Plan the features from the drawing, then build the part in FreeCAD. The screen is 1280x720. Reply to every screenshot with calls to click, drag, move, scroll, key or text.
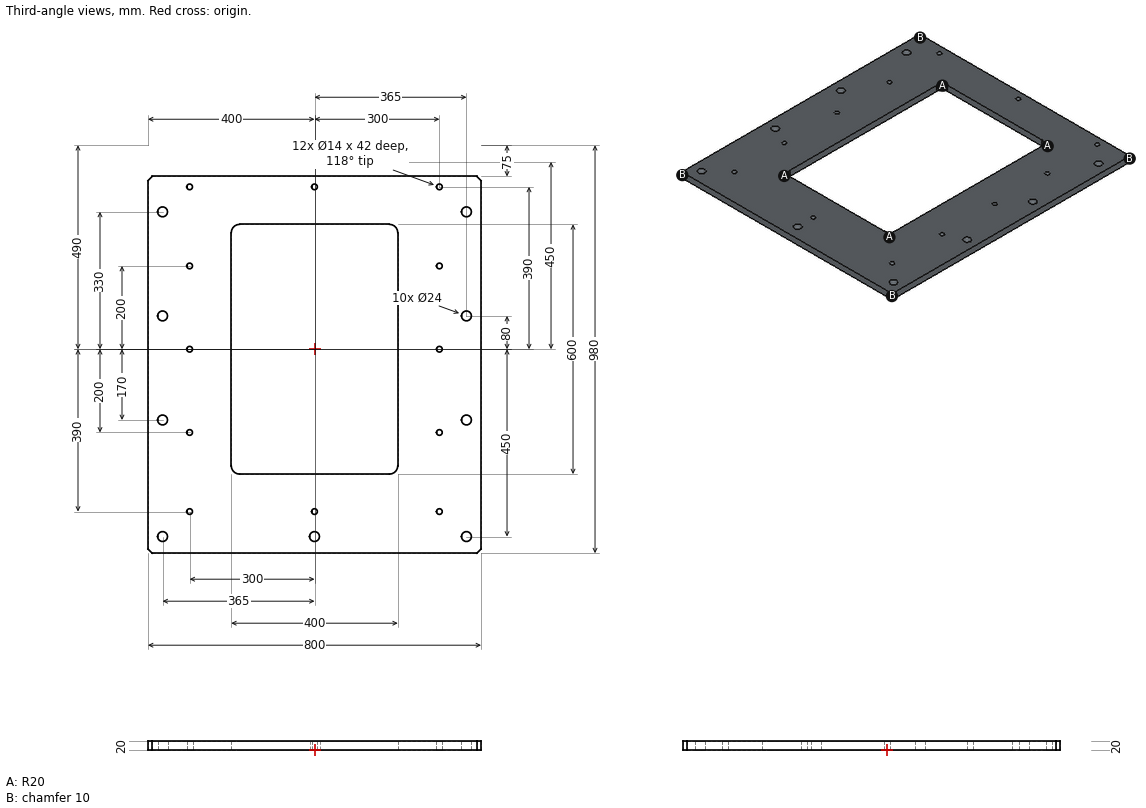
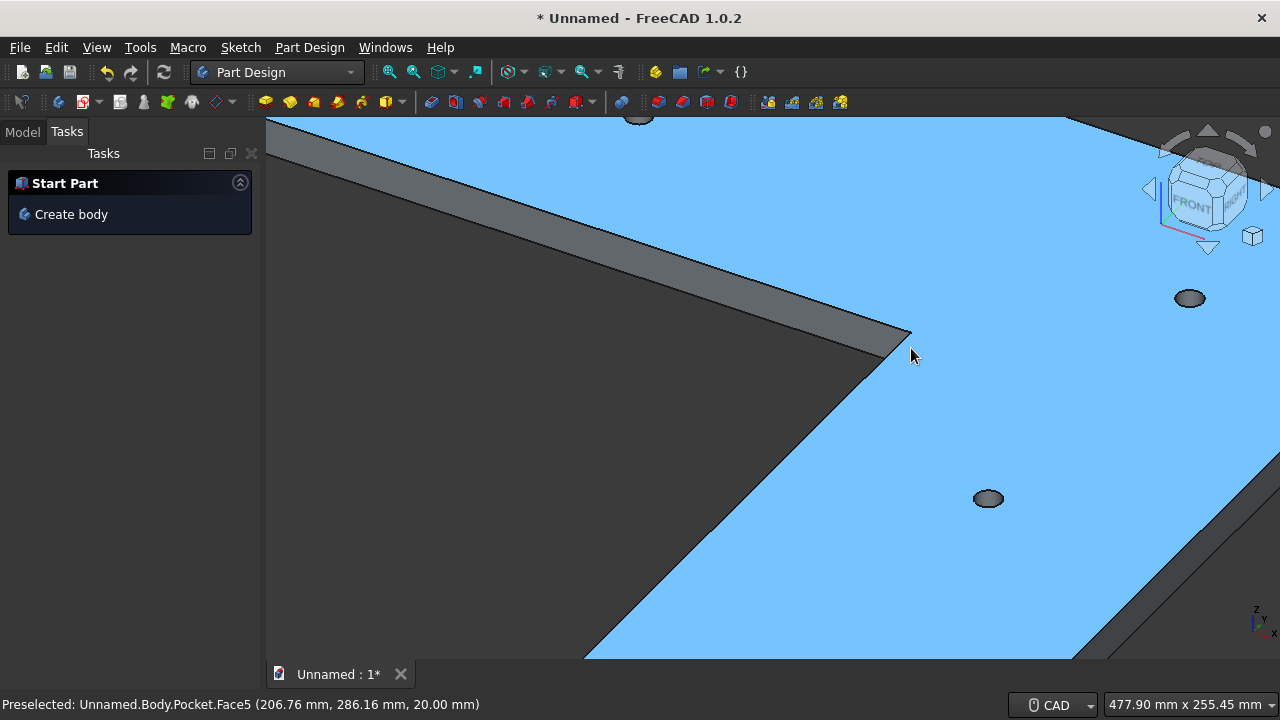
click(390, 72)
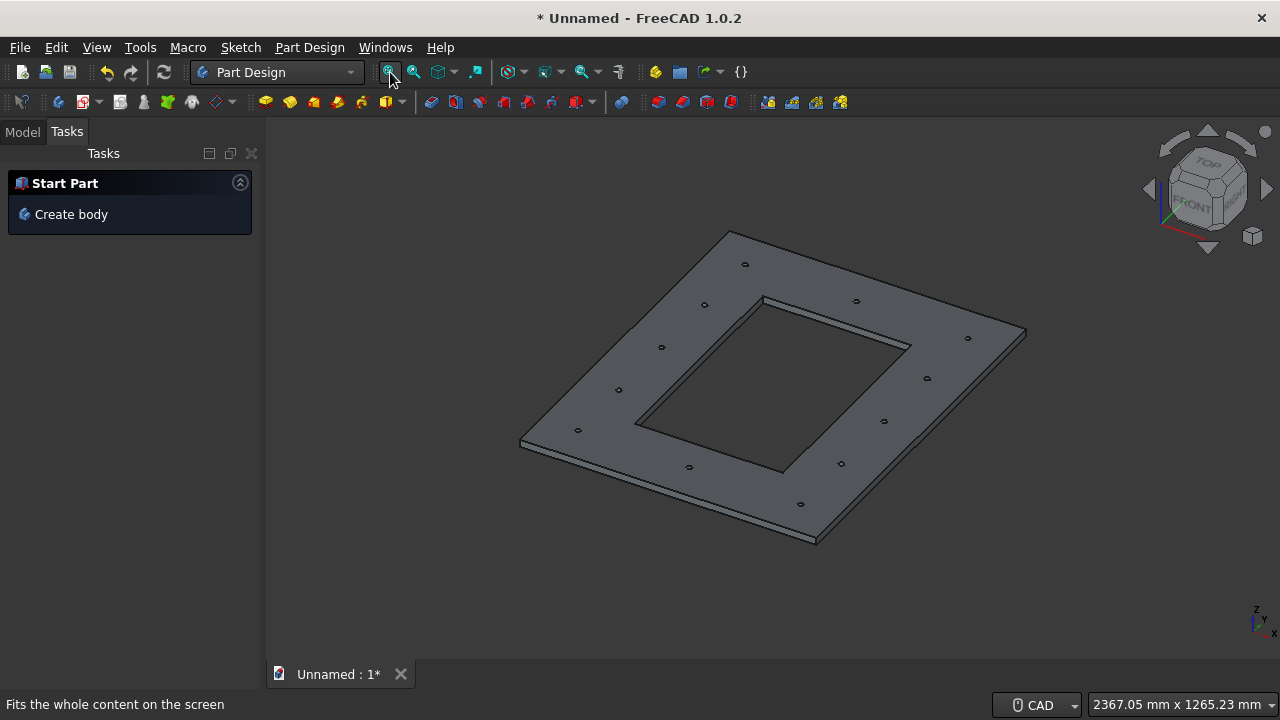
key(0)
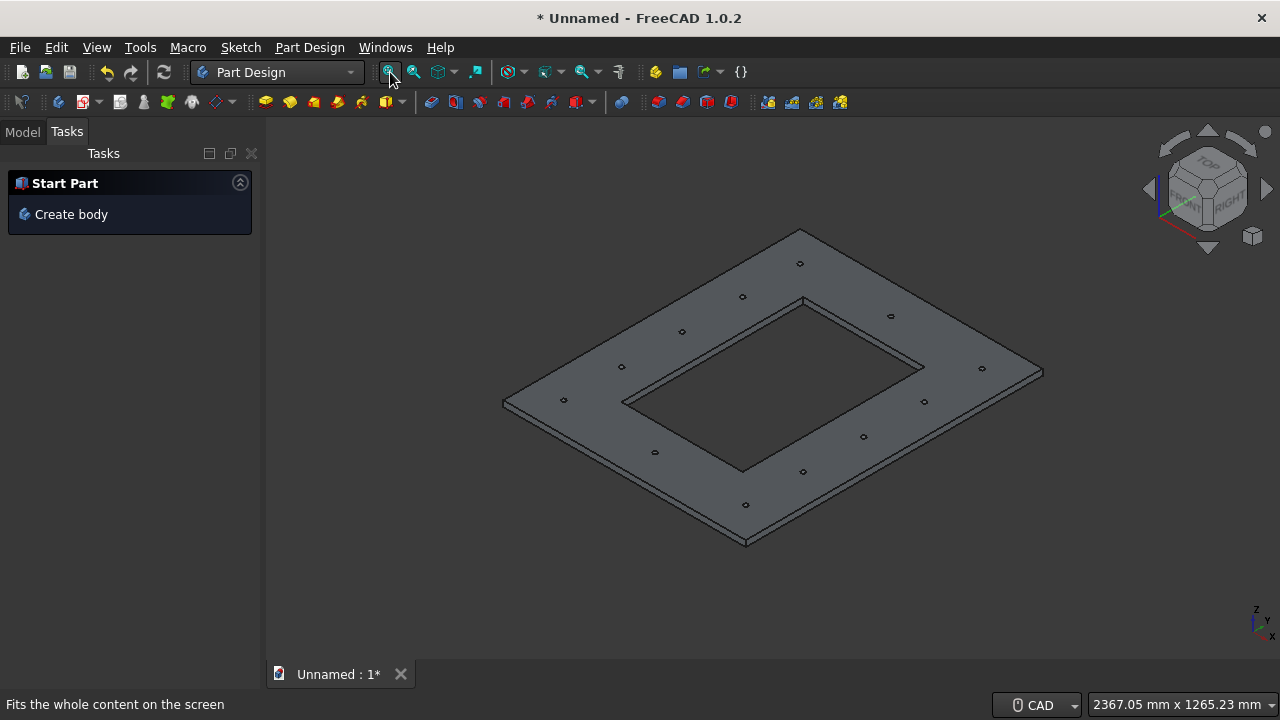
scroll(924, 370, up, 8)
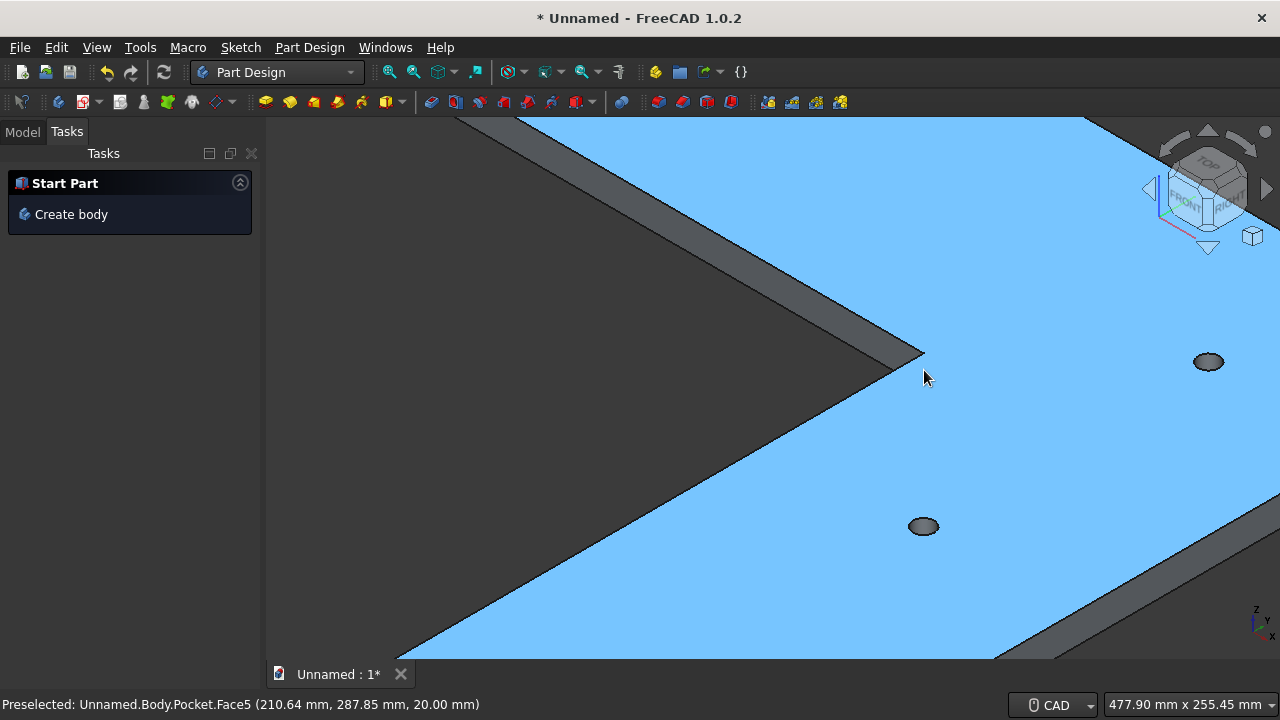
click(390, 72)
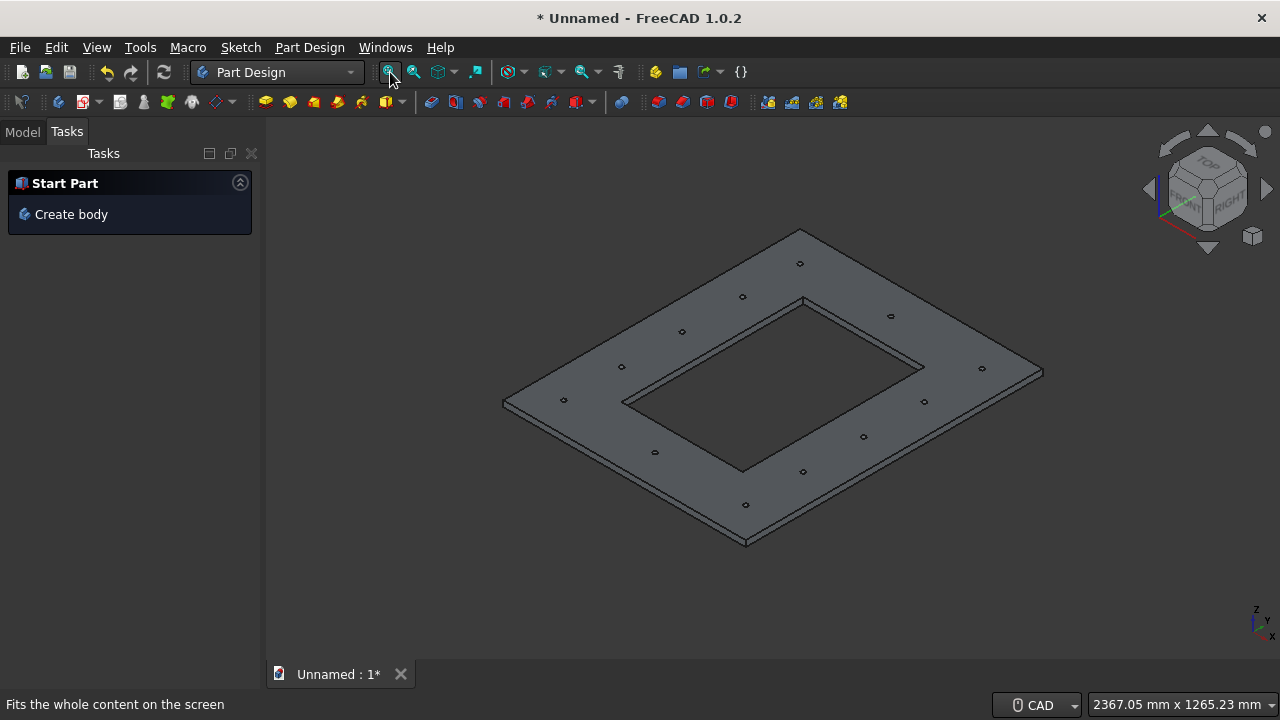
key(2)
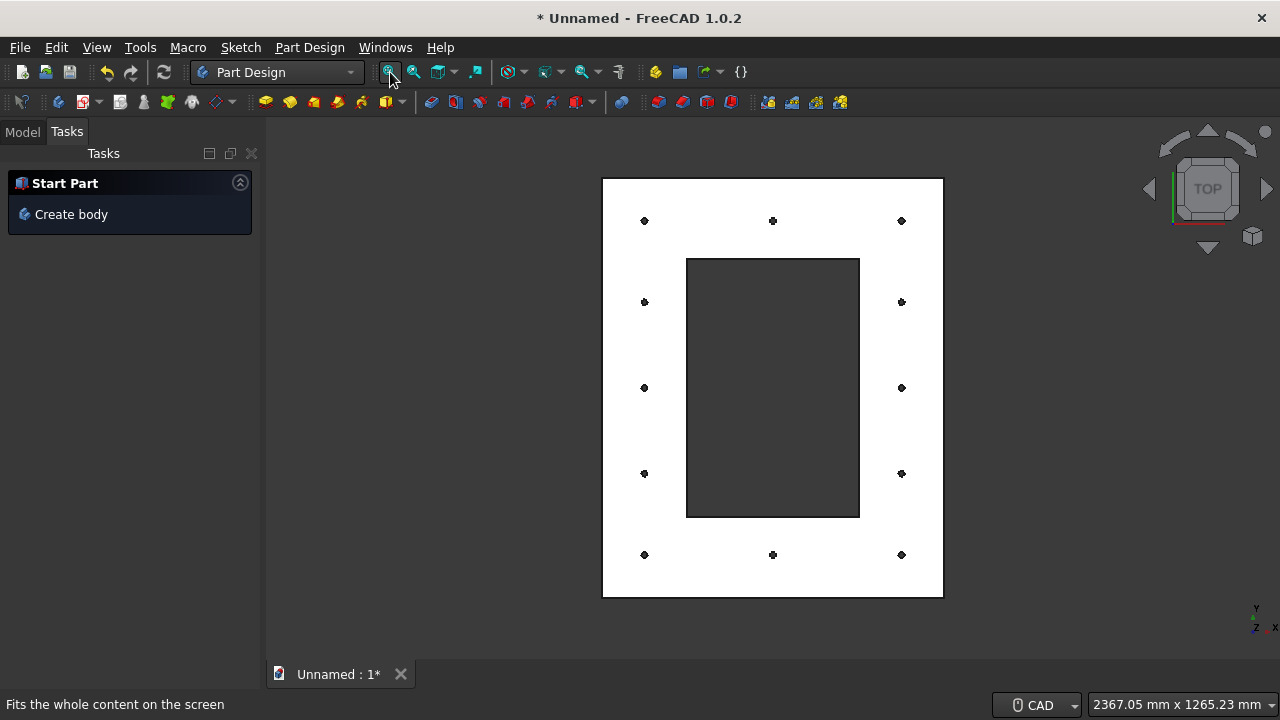
scroll(859, 258, up, 8)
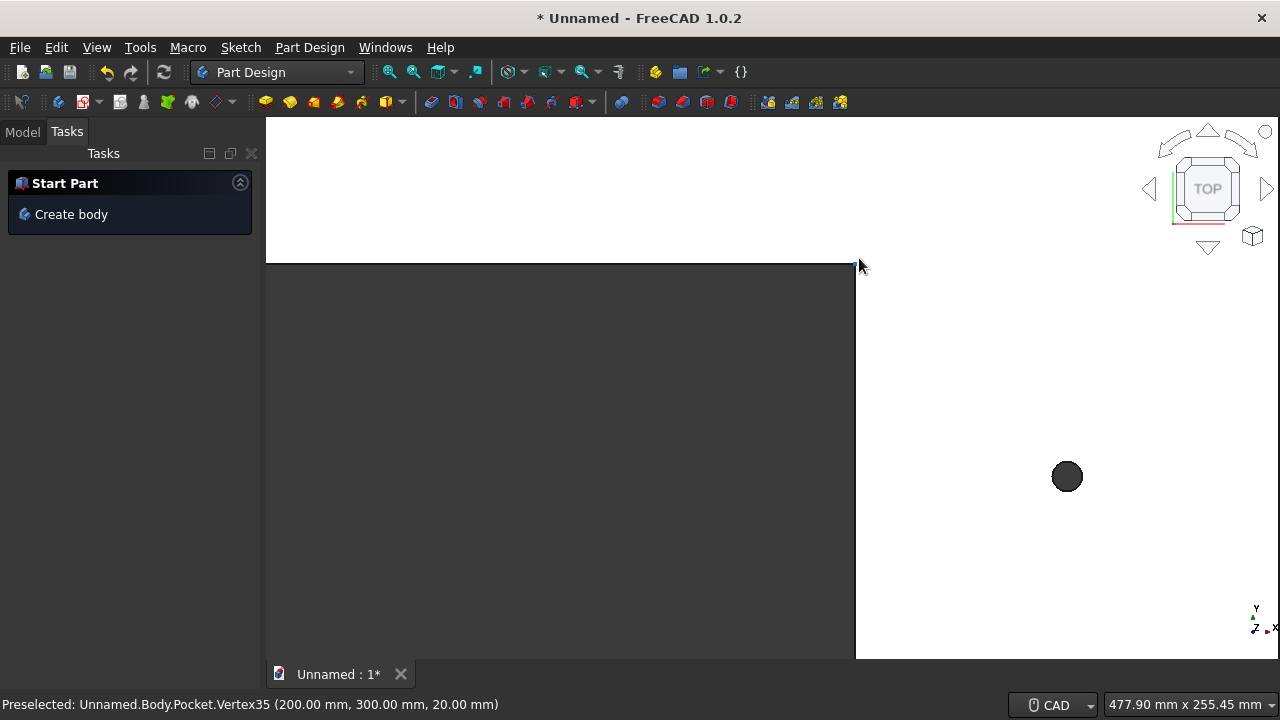
click(390, 72)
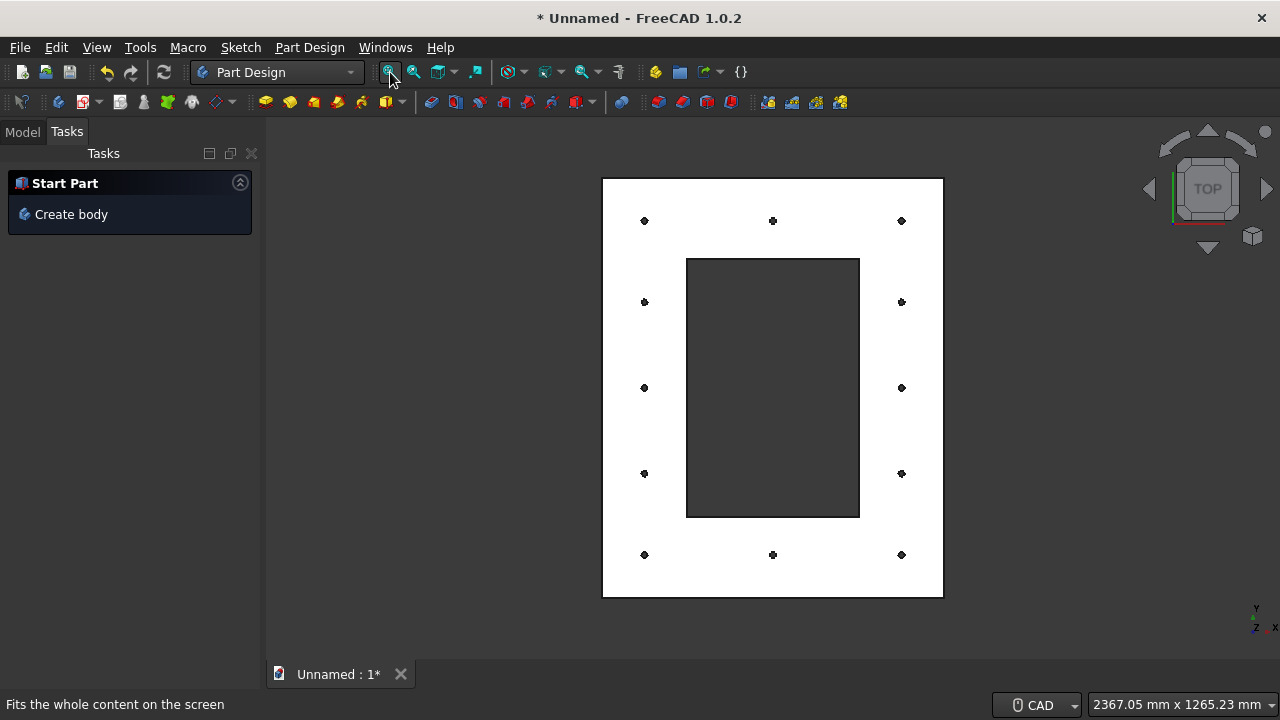
key(1)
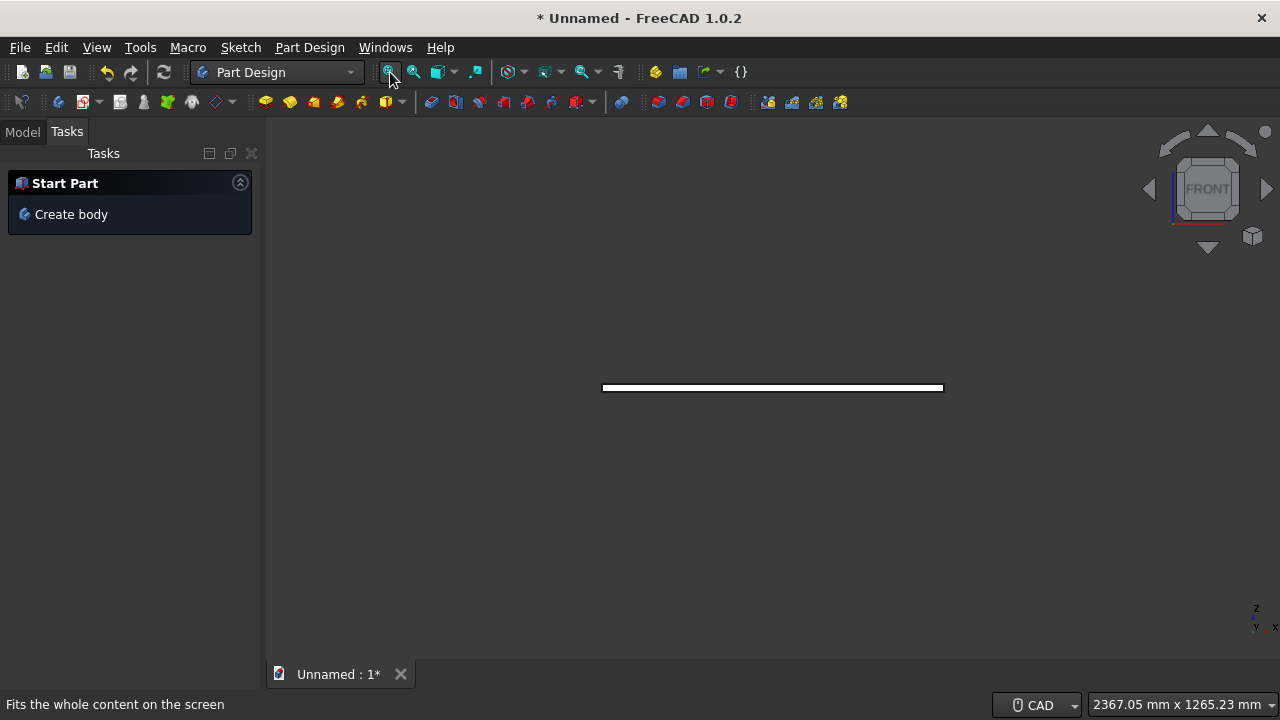
click(390, 72)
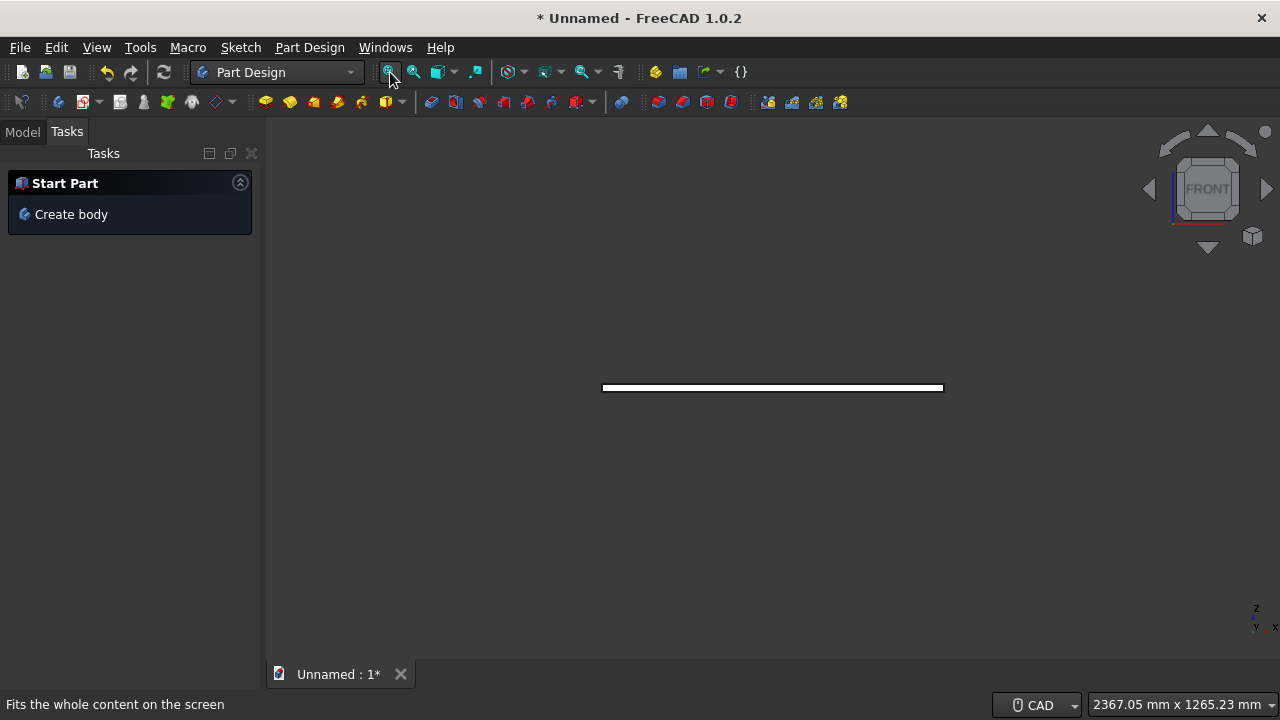
scroll(859, 387, up, 8)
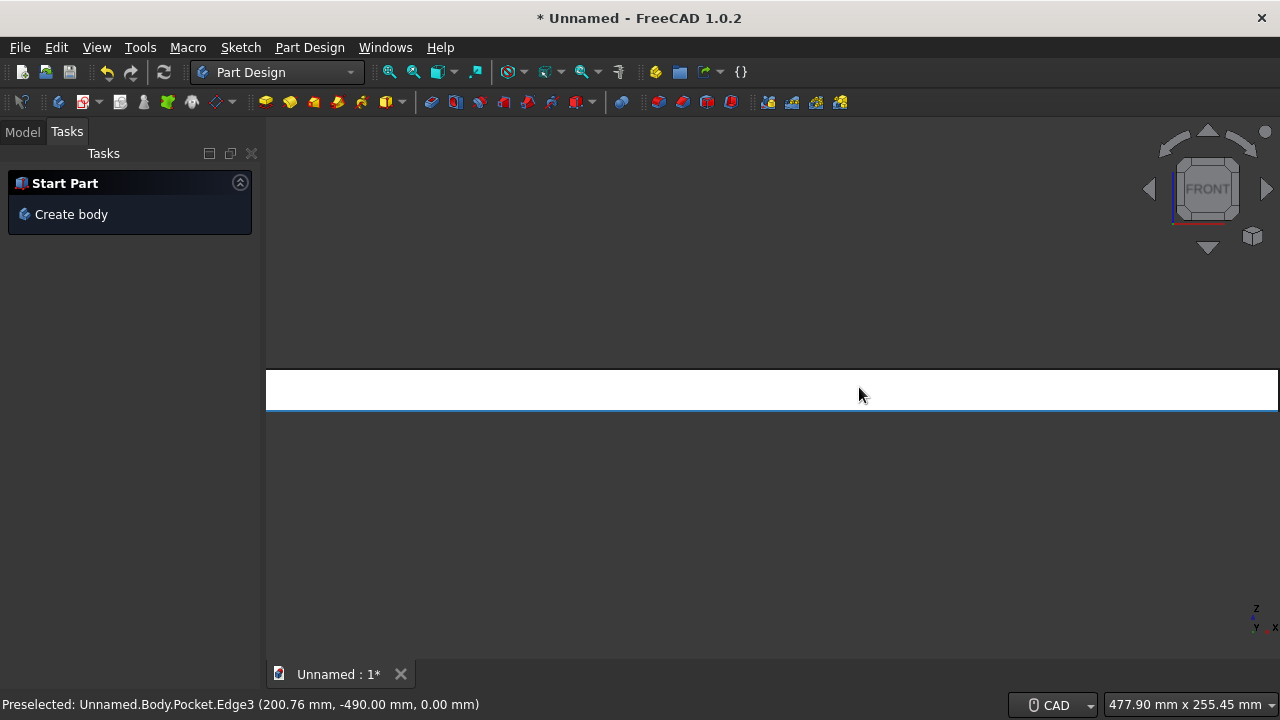
click(390, 72)